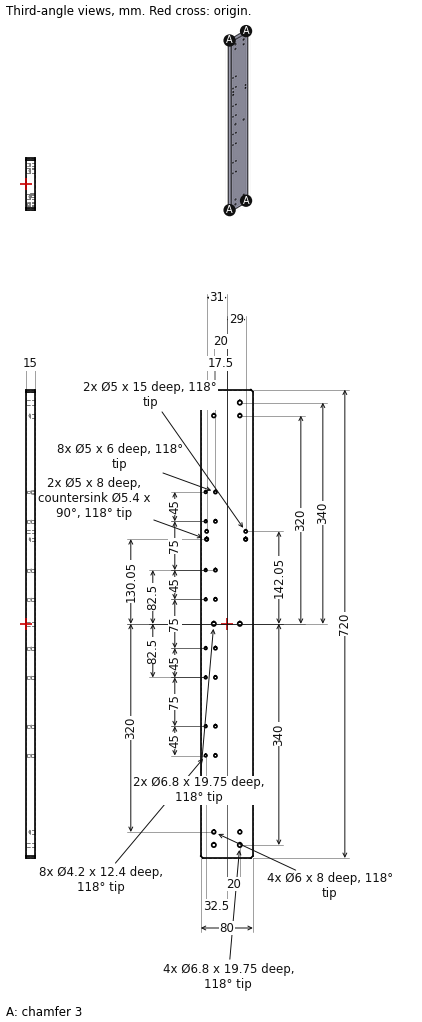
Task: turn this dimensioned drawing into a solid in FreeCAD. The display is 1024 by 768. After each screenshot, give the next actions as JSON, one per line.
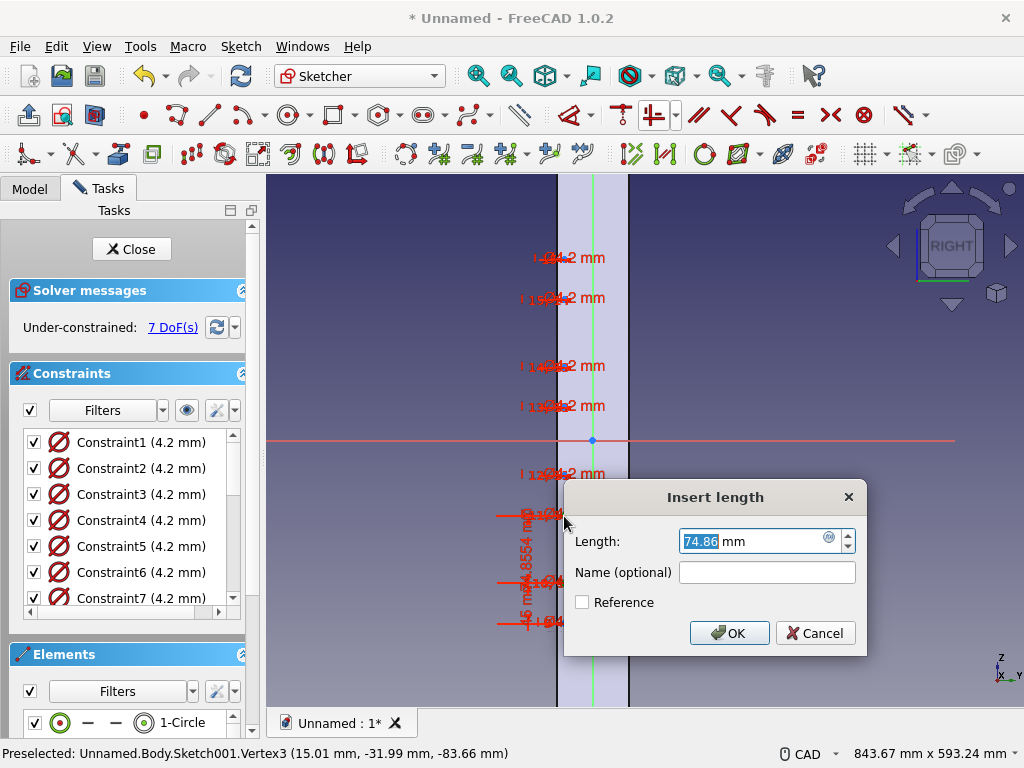
{"action": "type", "text": "75"}
{"action": "key", "text": "Return"}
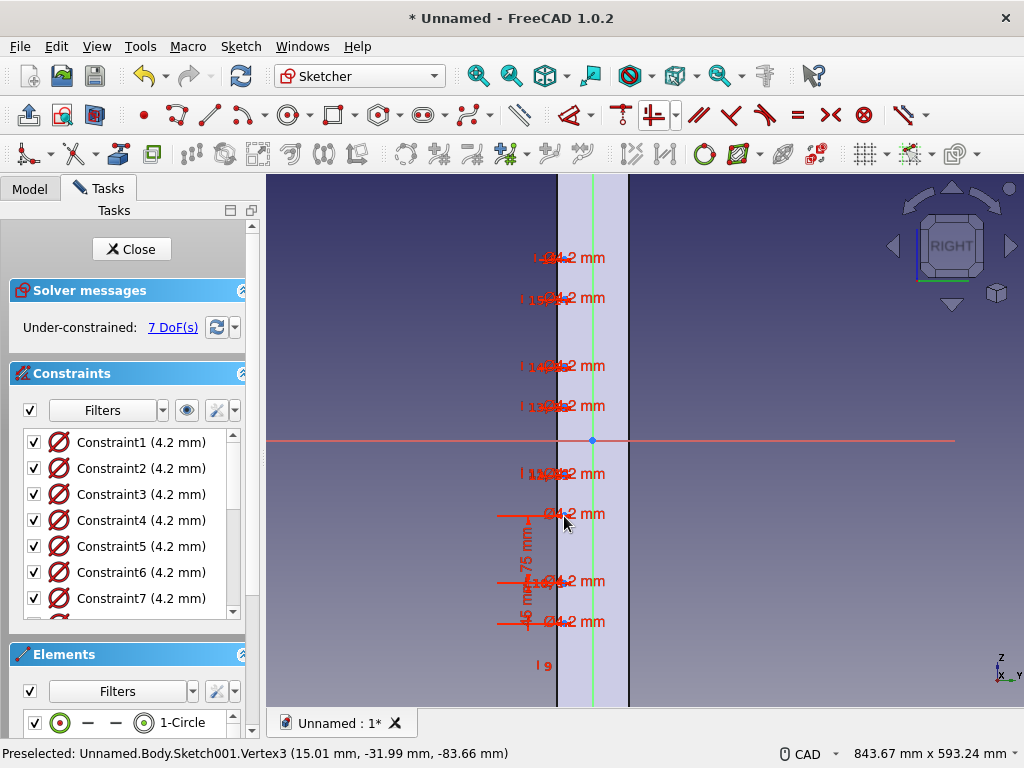
{"action": "left_click", "coordinate": [564, 516]}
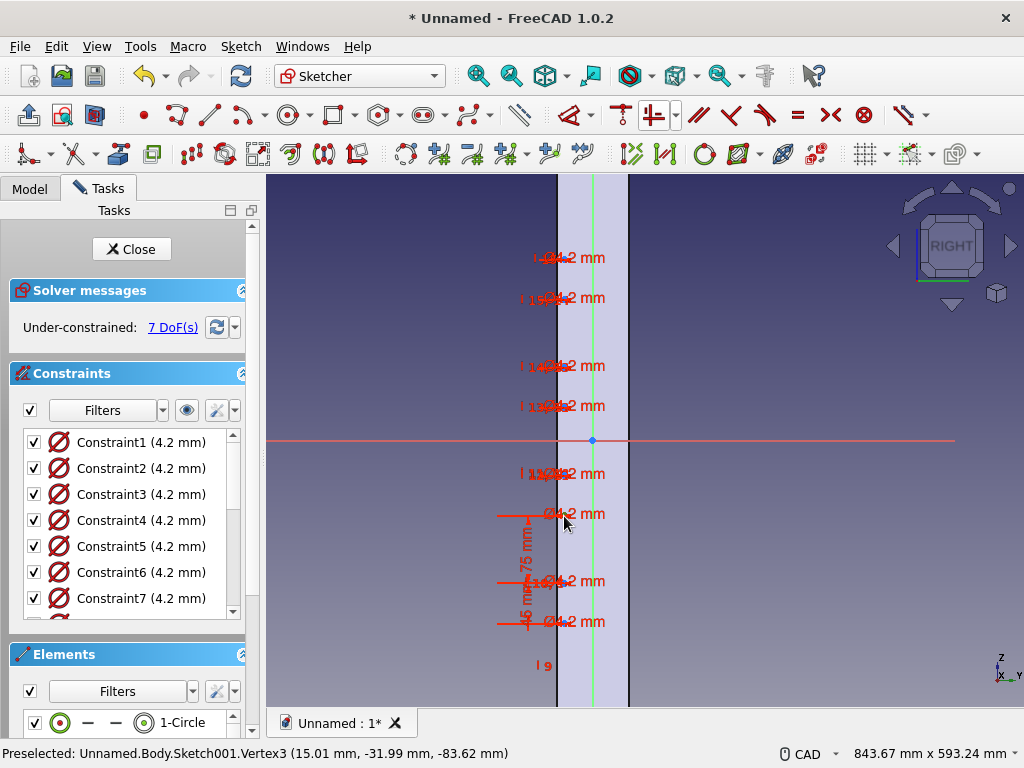
{"action": "left_click", "coordinate": [564, 476]}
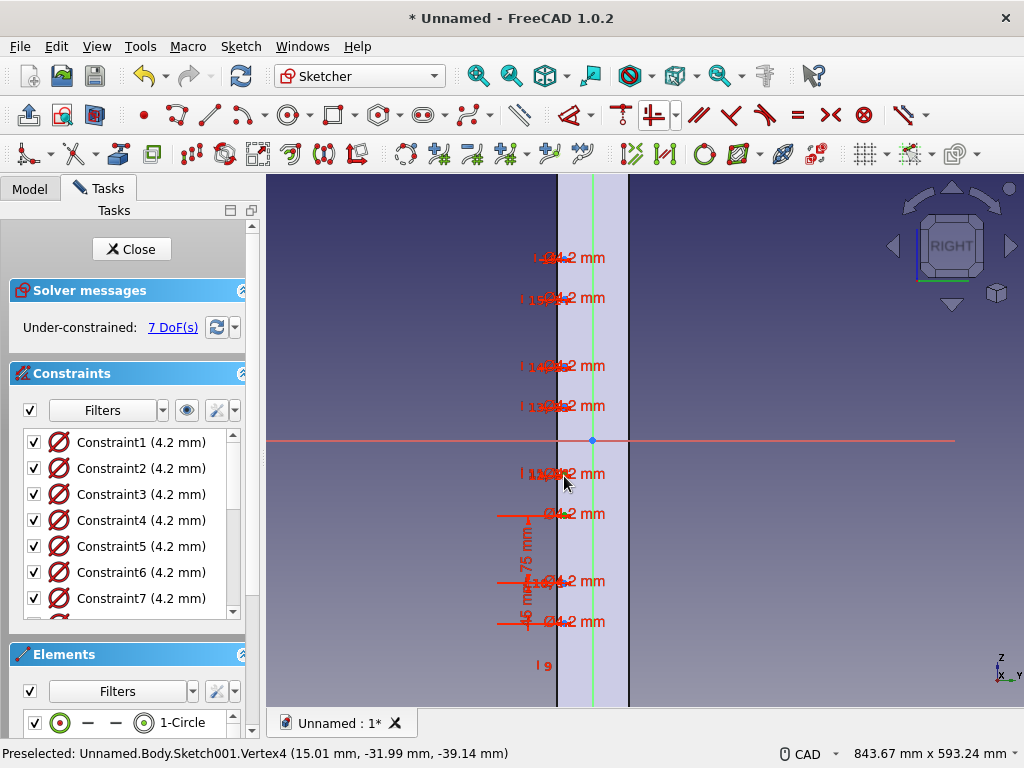
{"action": "key", "text": "i"}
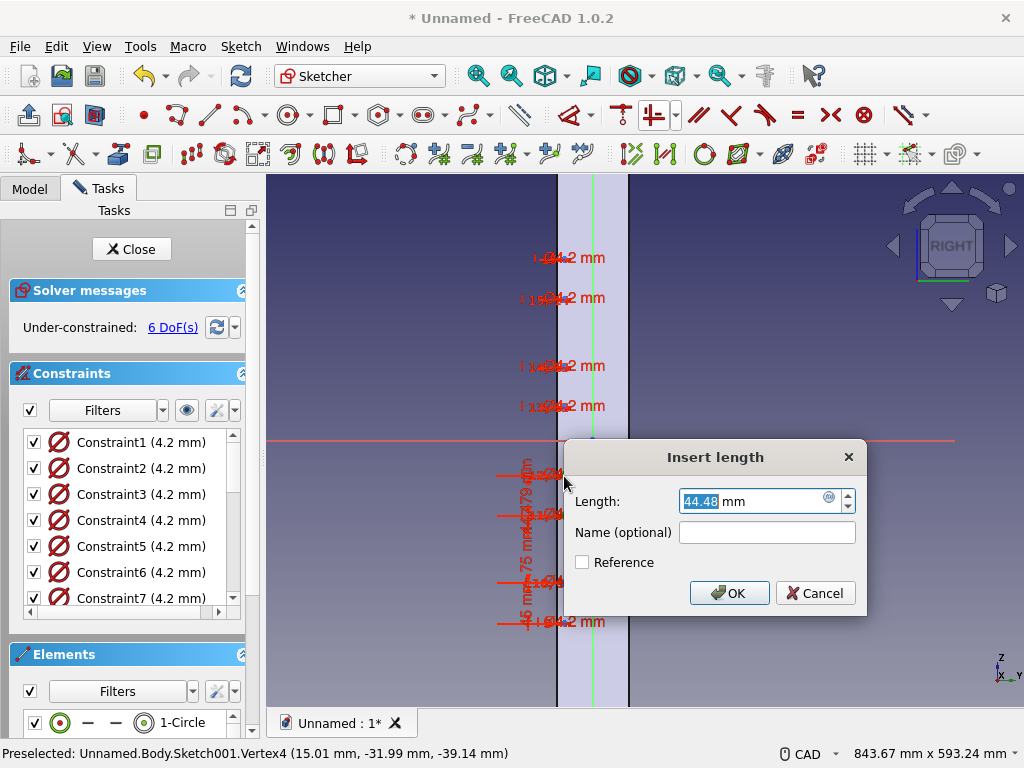
{"action": "type", "text": "45"}
{"action": "key", "text": "Return"}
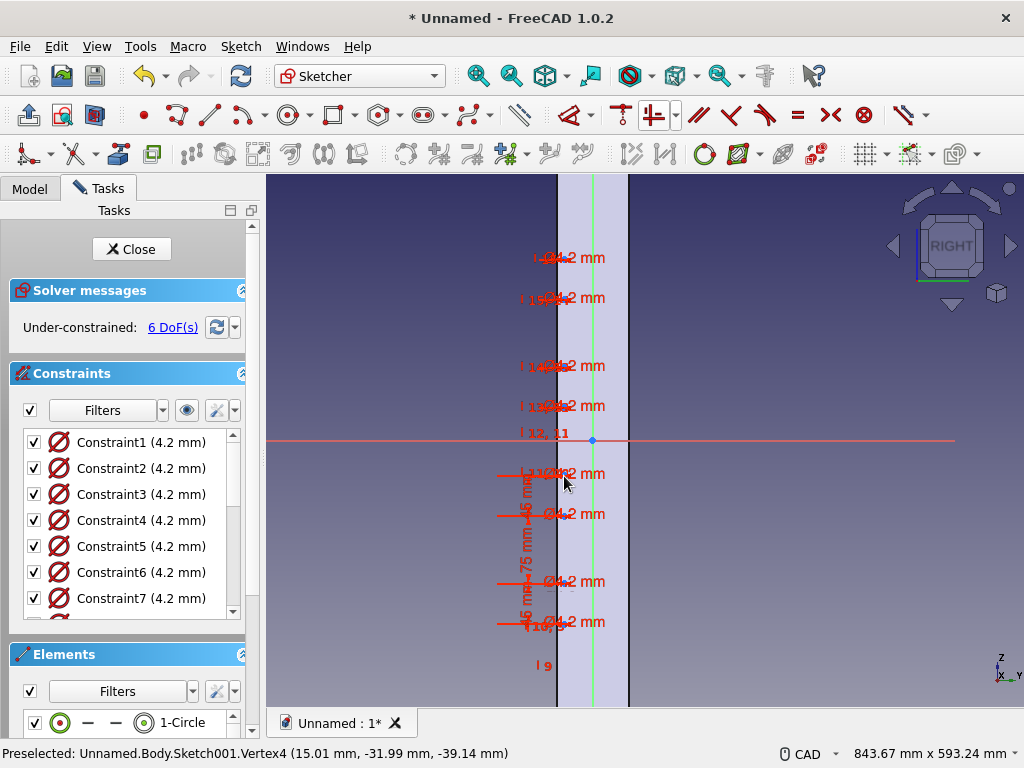
{"action": "left_click", "coordinate": [564, 476]}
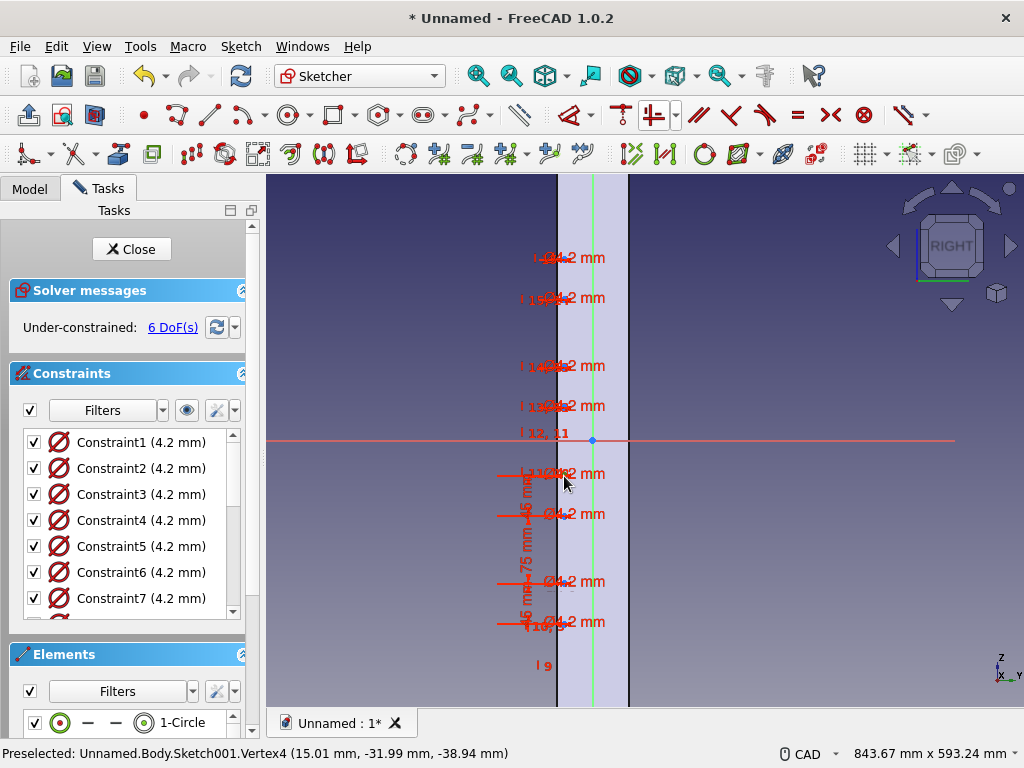
{"action": "left_click", "coordinate": [564, 408]}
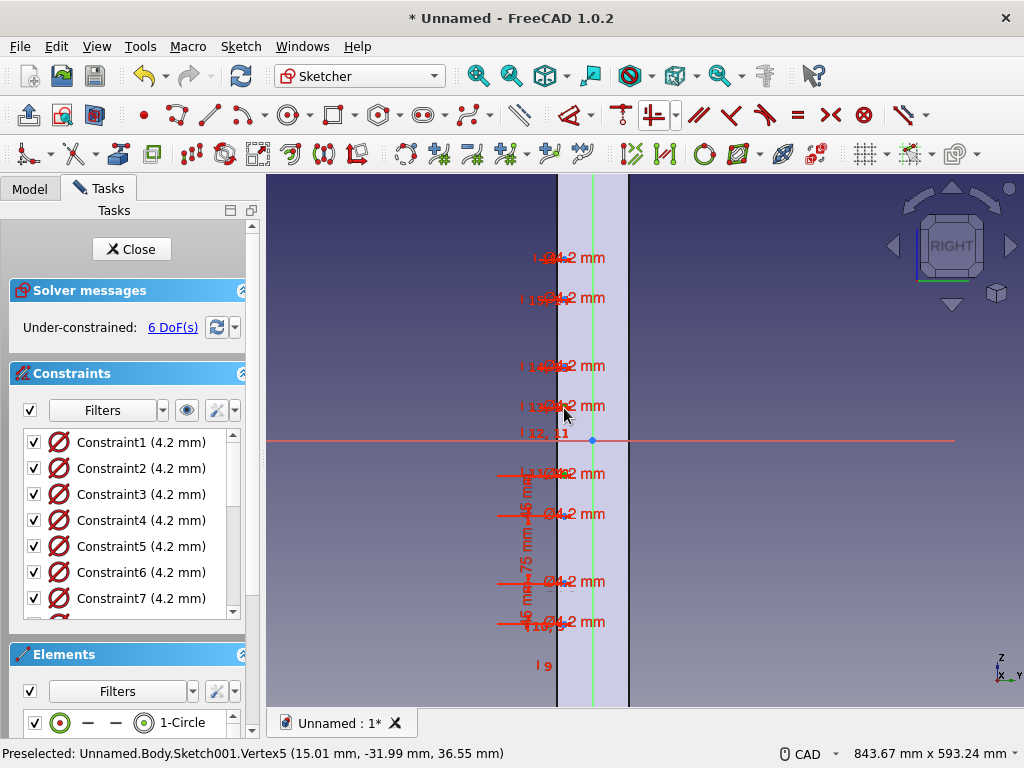
{"action": "left_click", "coordinate": [590, 116]}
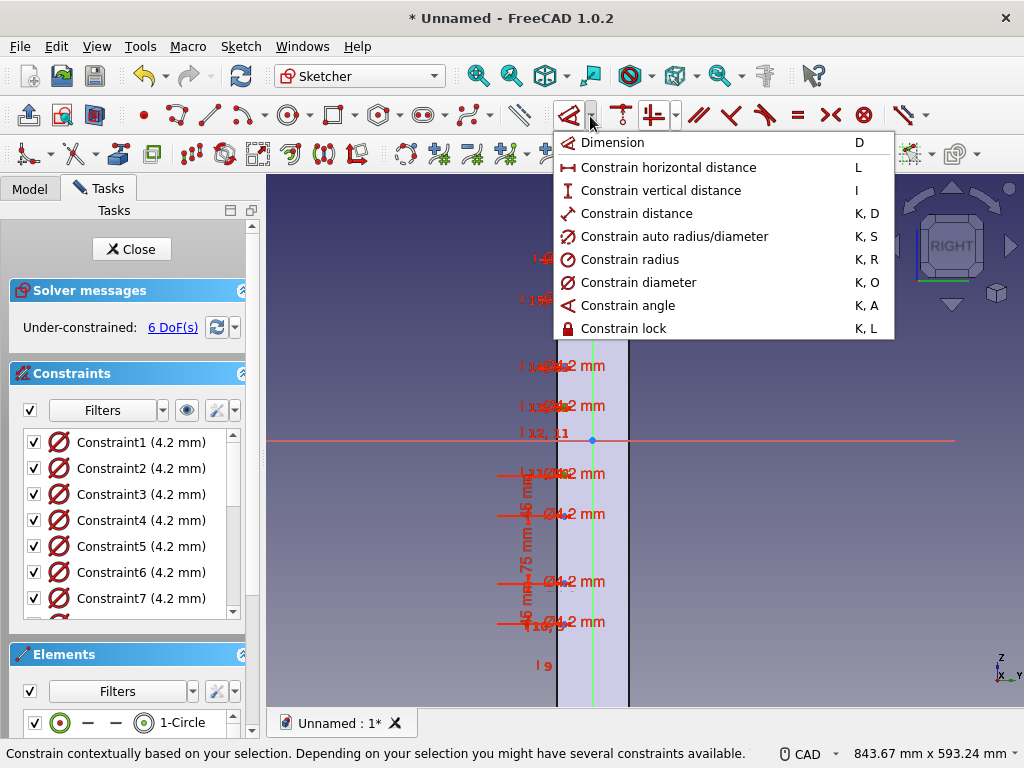
{"action": "left_click", "coordinate": [724, 190]}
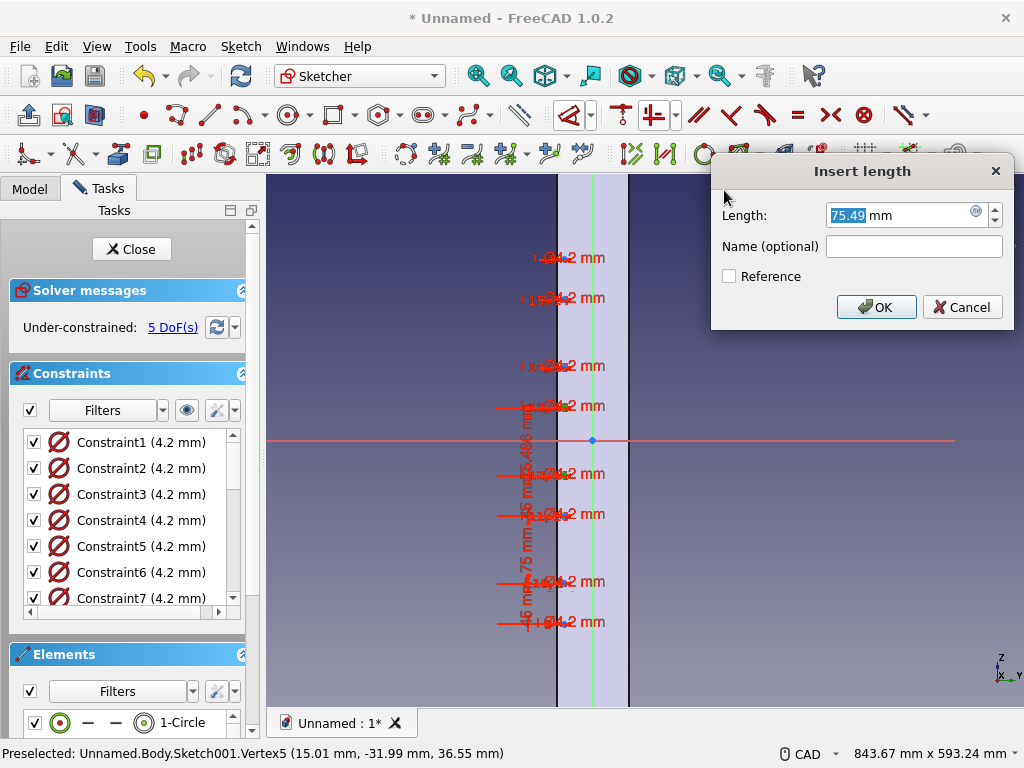
{"action": "type", "text": "75"}
{"action": "key", "text": "Return"}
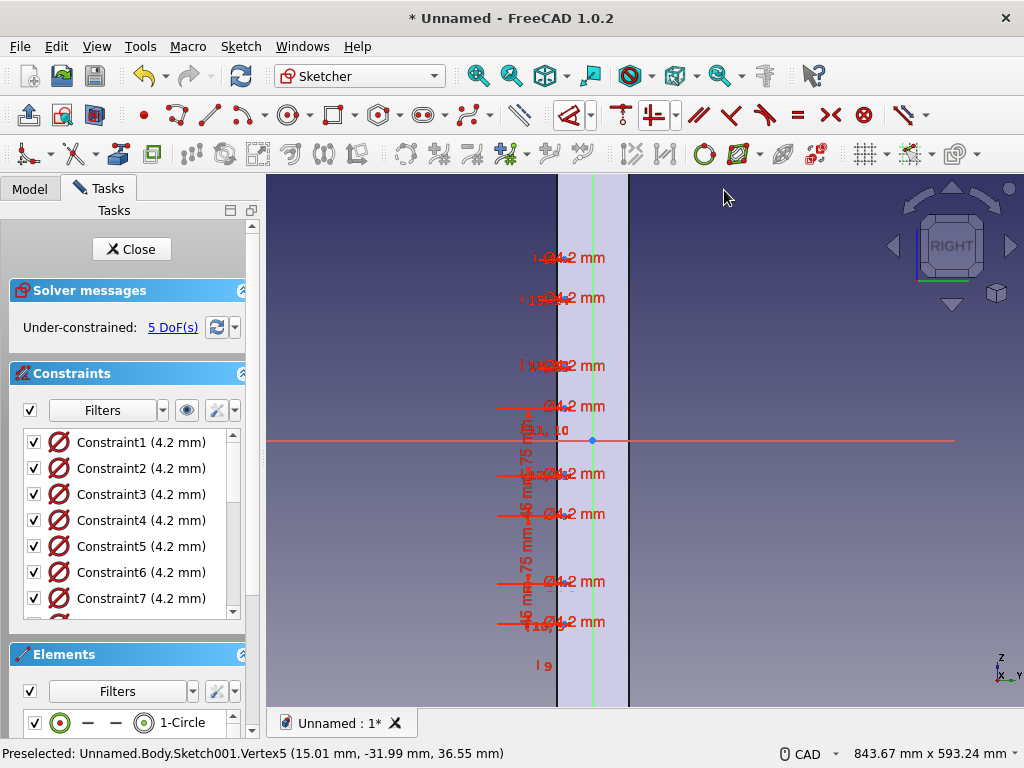
{"action": "left_click", "coordinate": [564, 408]}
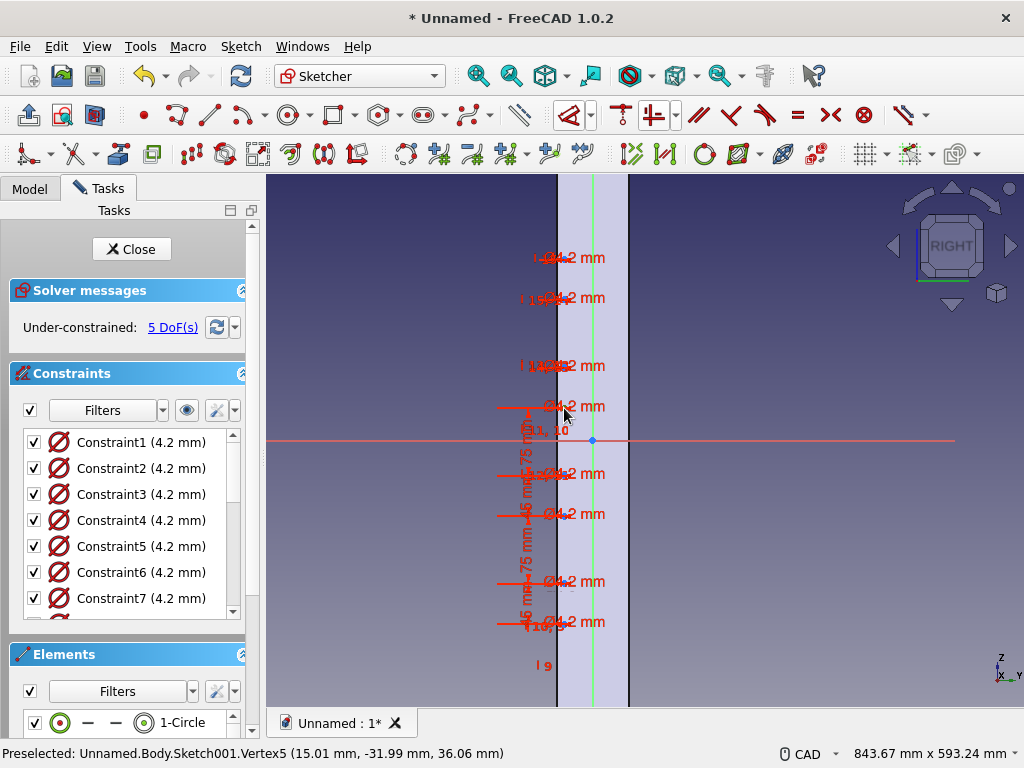
{"action": "left_click", "coordinate": [564, 368]}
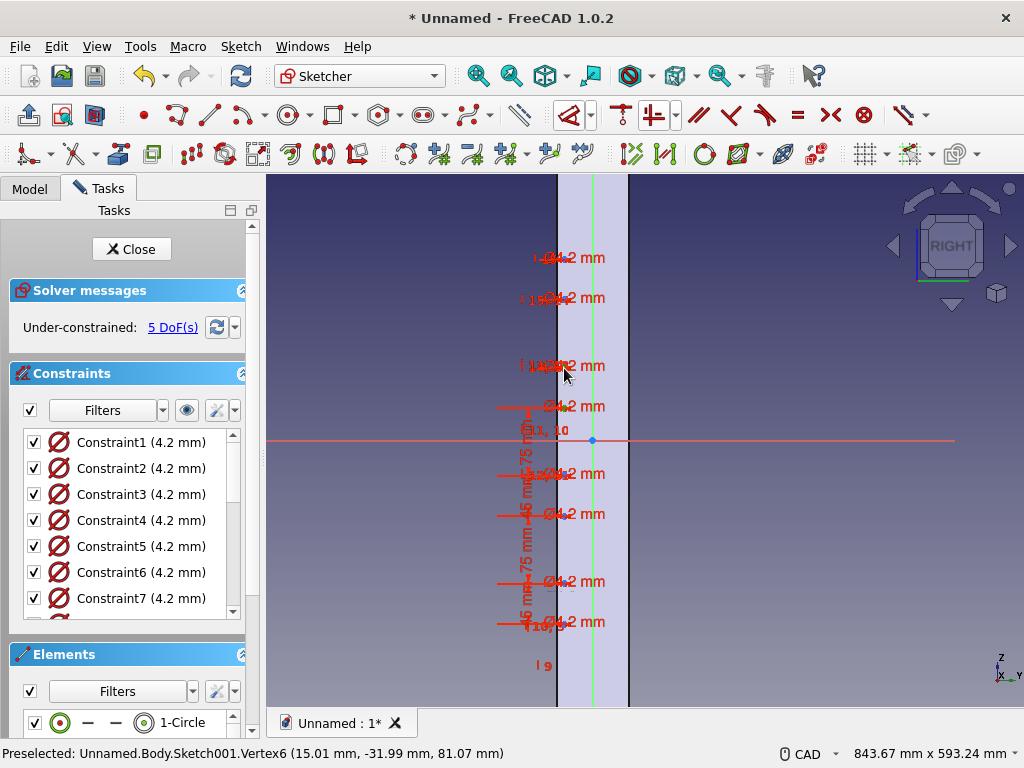
{"action": "key", "text": "i"}